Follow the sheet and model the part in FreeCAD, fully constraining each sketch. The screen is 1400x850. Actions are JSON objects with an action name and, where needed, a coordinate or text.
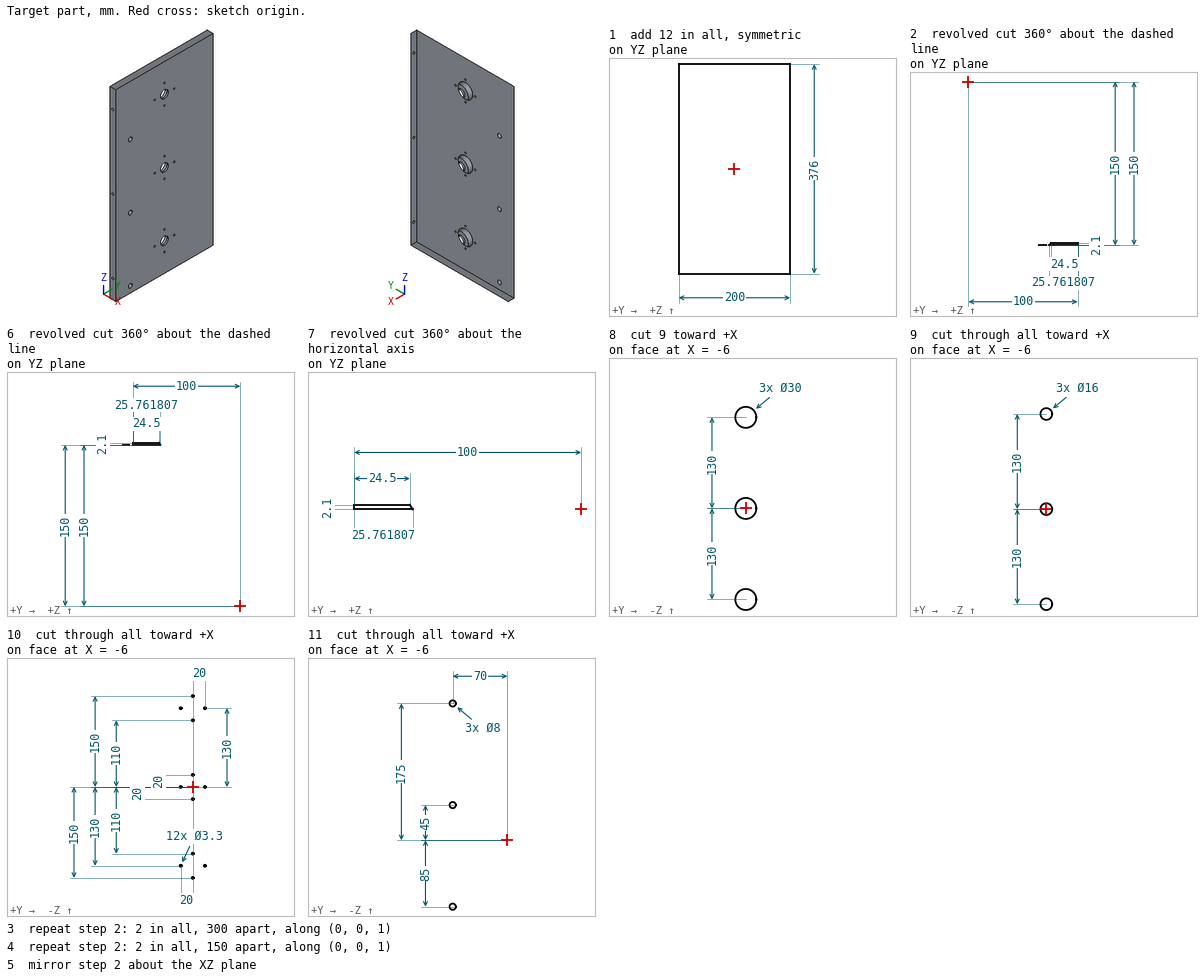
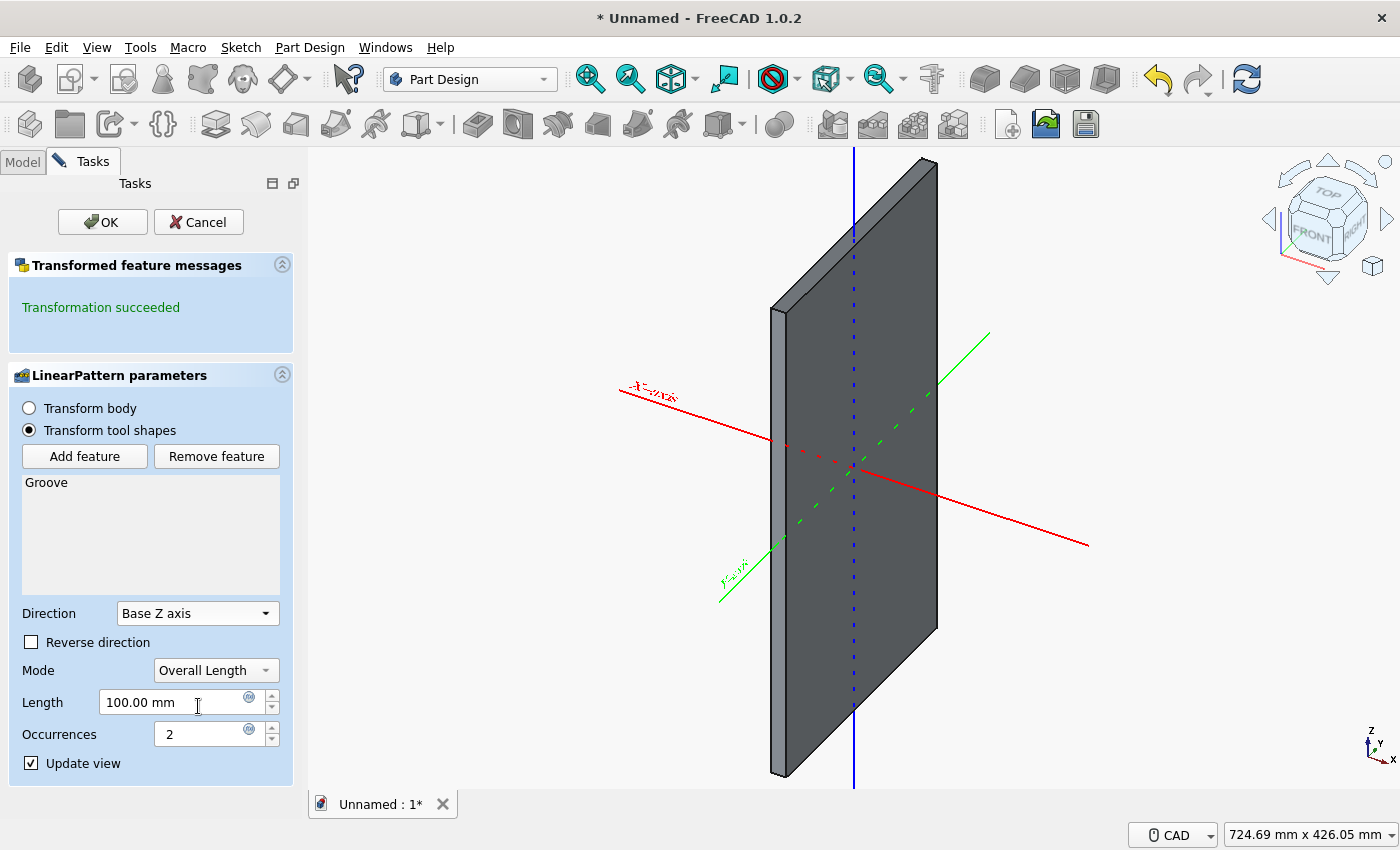
{"action": "left_click", "coordinate": [217, 670]}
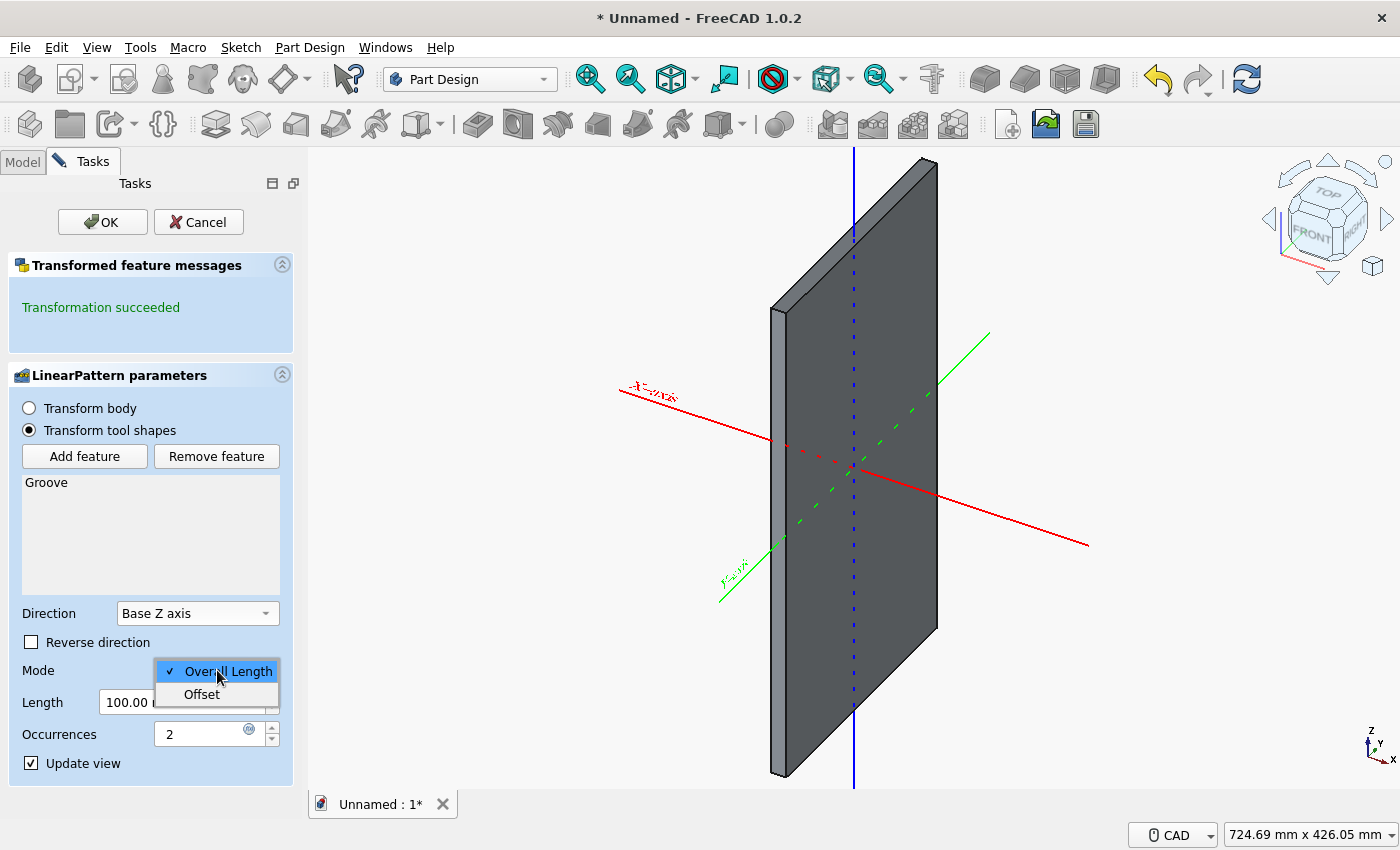
{"action": "left_click", "coordinate": [216, 694]}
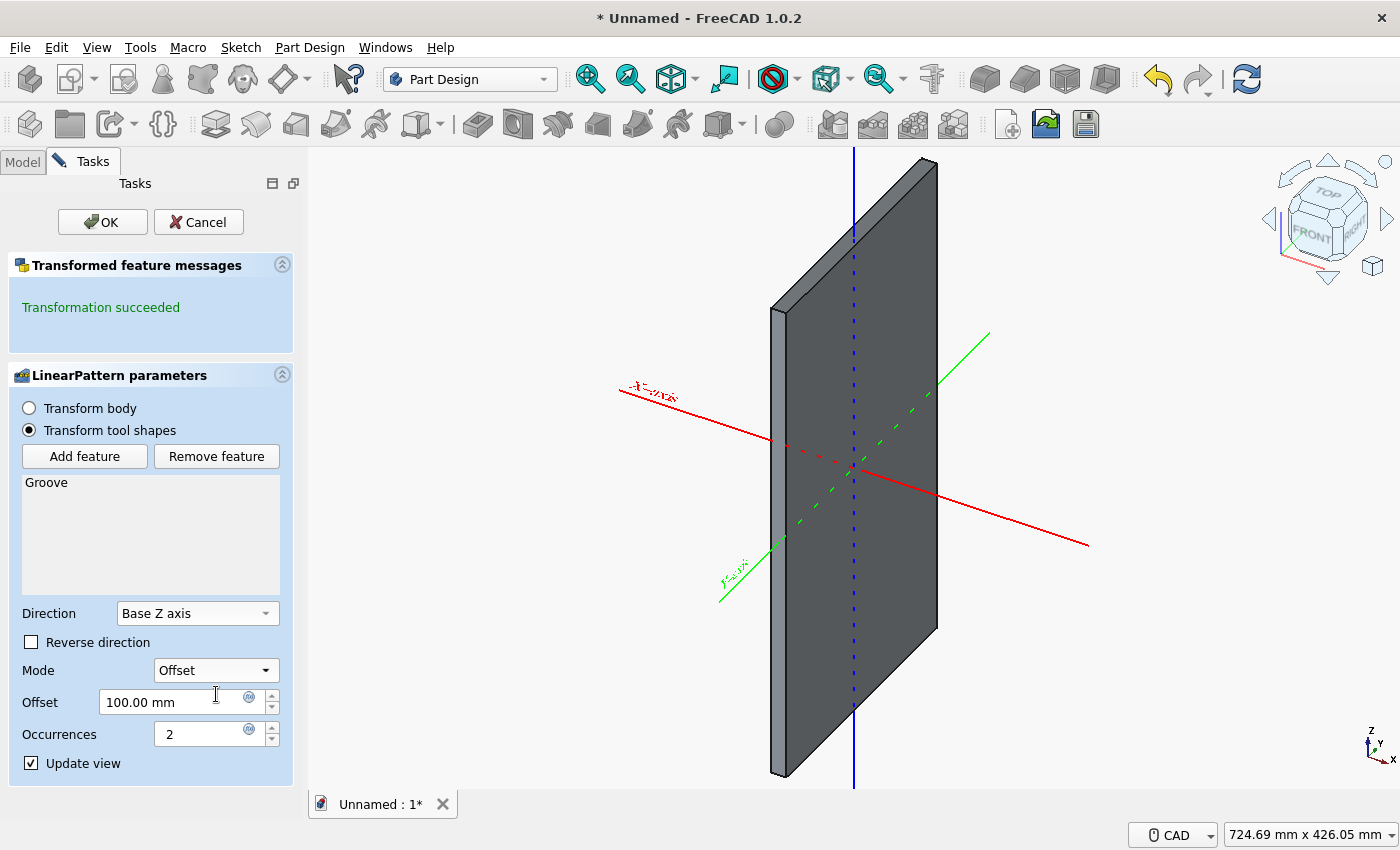
{"action": "triple_click", "coordinate": [182, 702]}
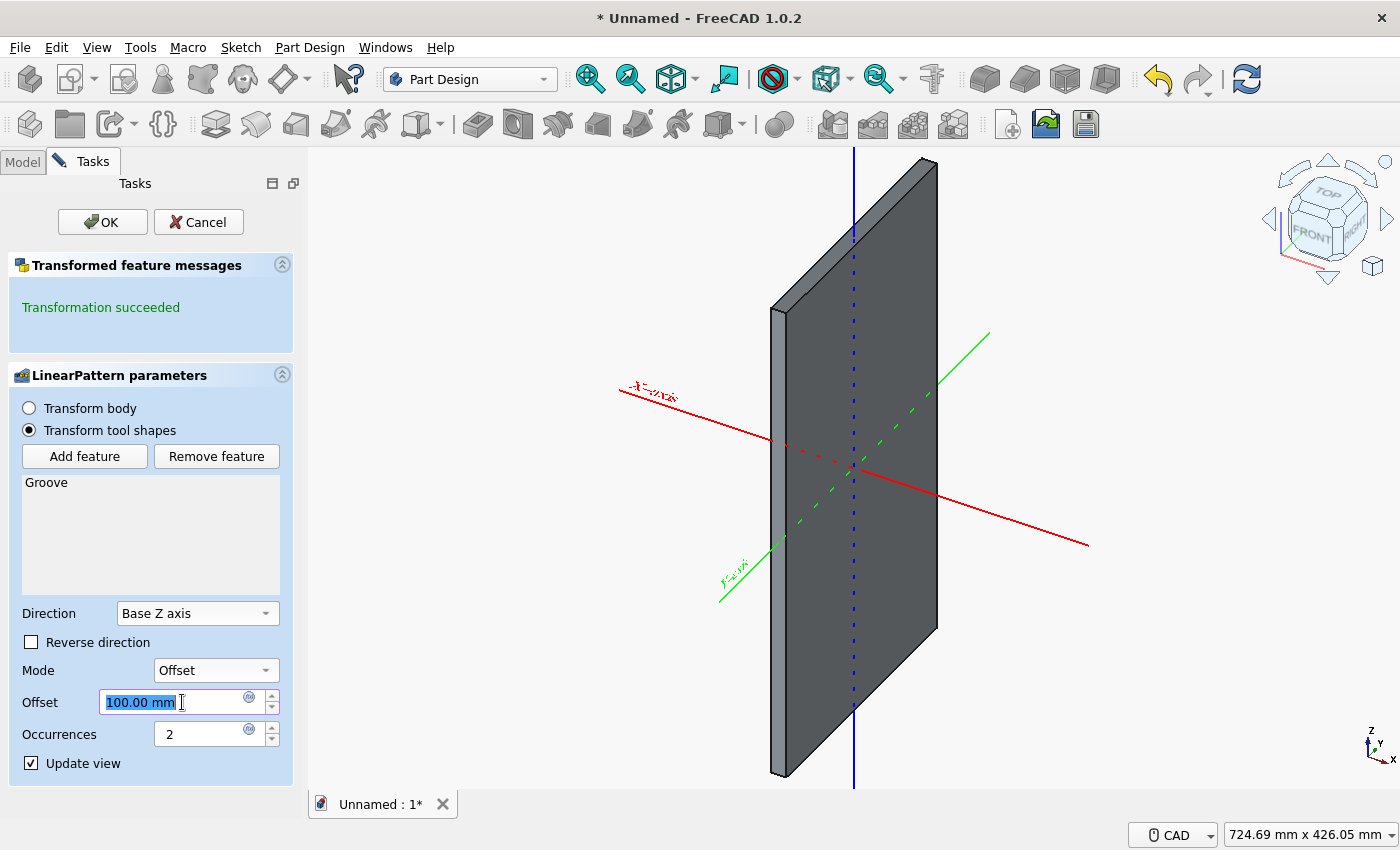
{"action": "type", "text": "300"}
{"action": "key", "text": "Tab"}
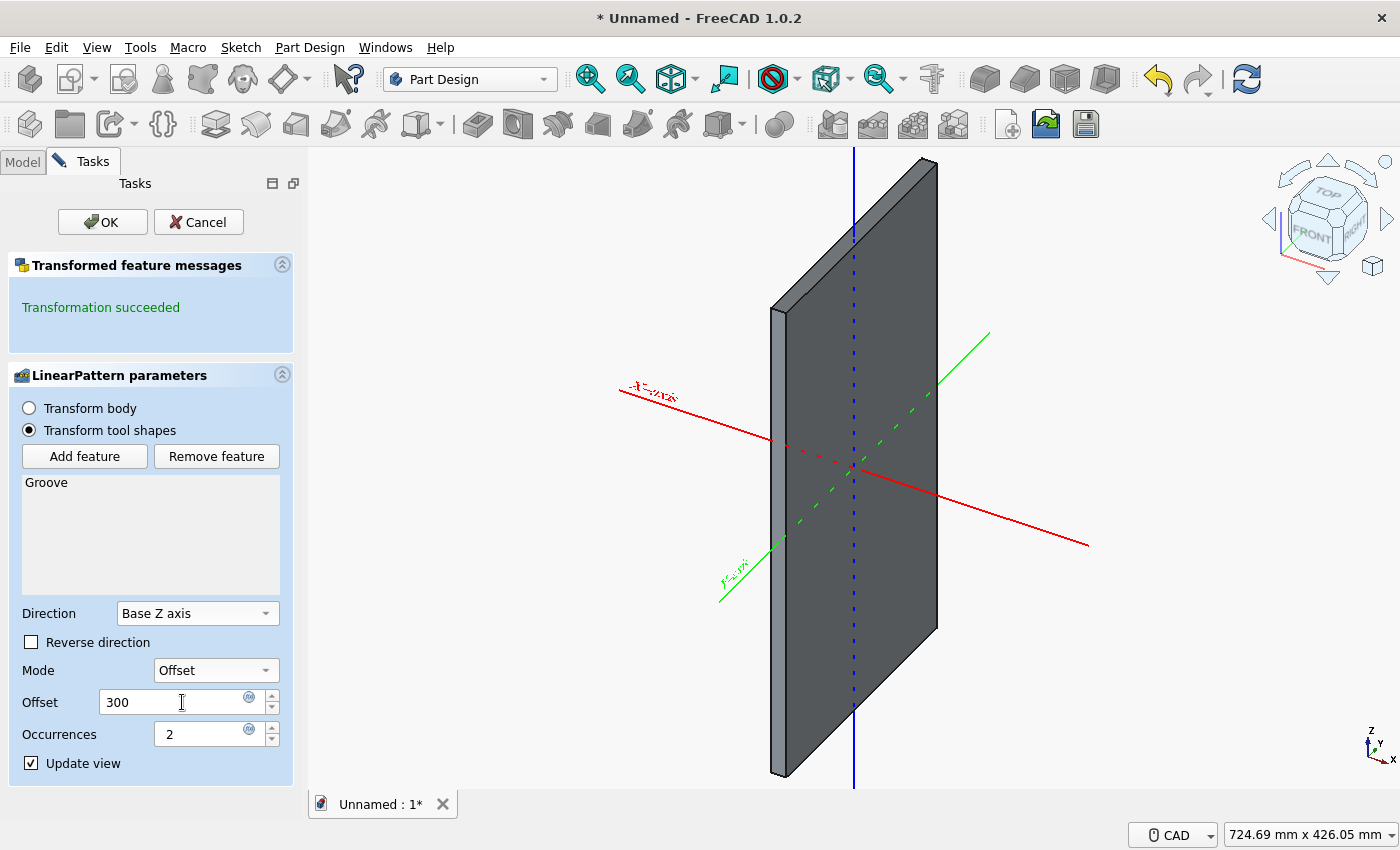
{"action": "triple_click", "coordinate": [209, 734]}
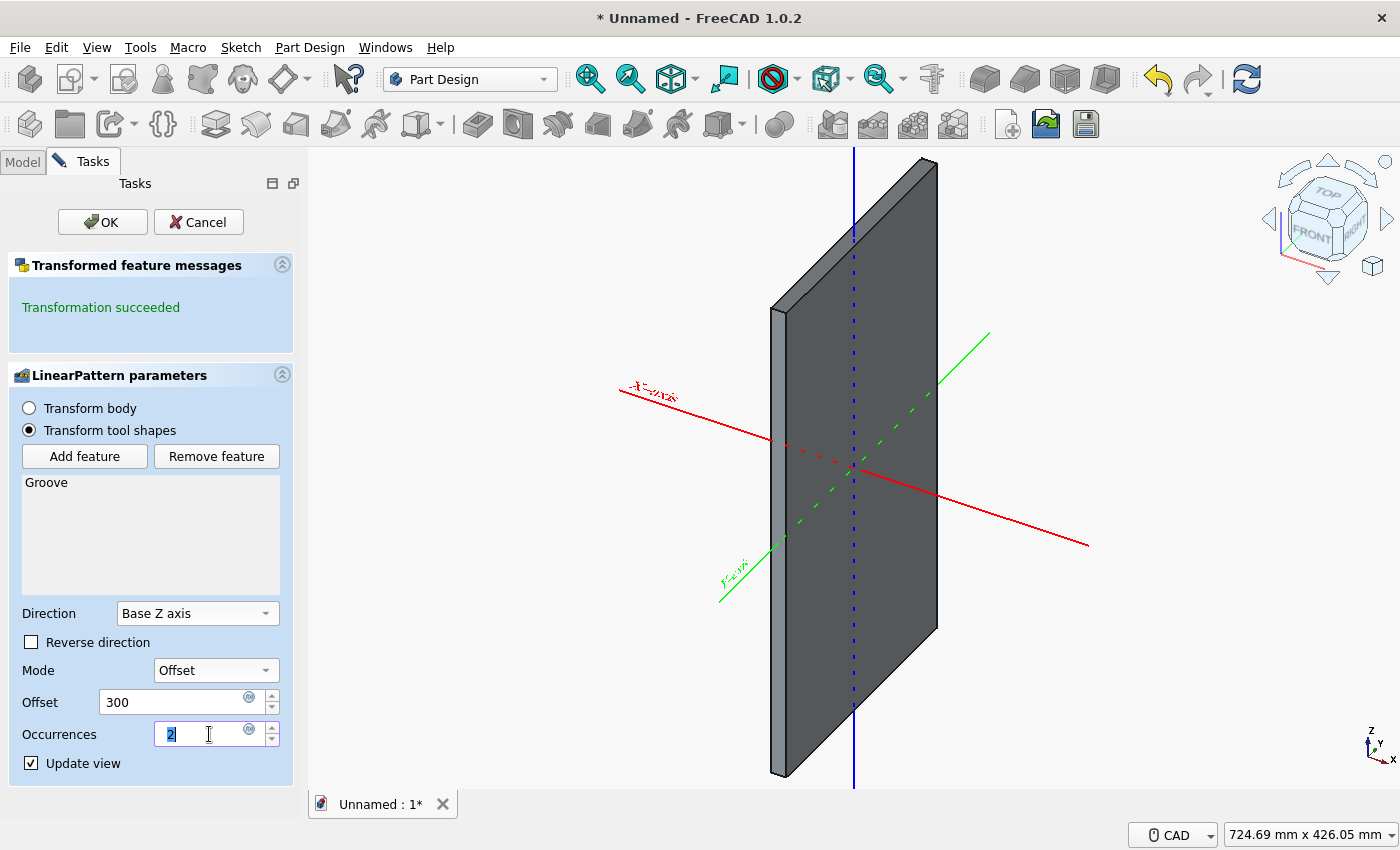
{"action": "type", "text": "2"}
{"action": "key", "text": "Tab"}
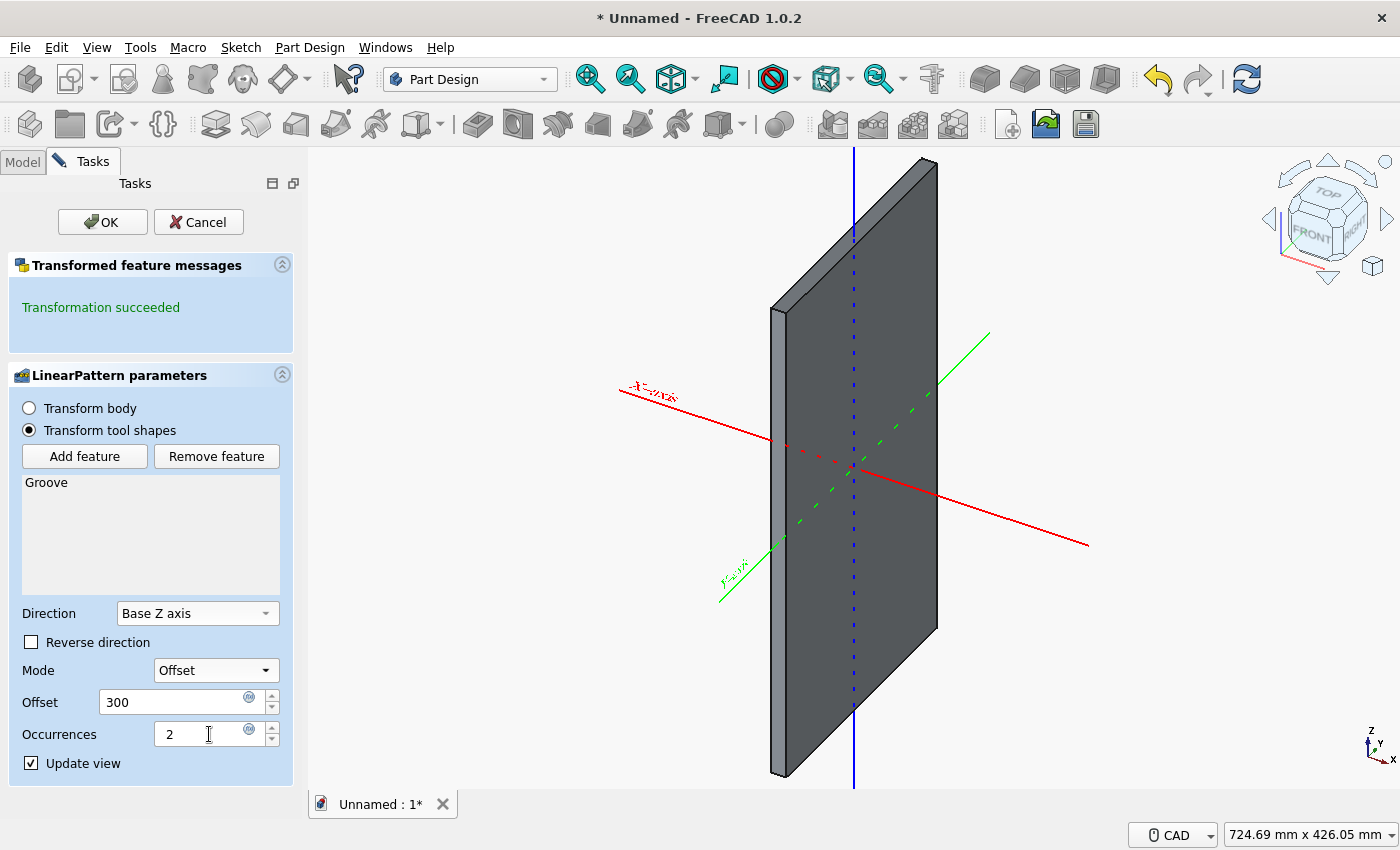
{"action": "left_click", "coordinate": [103, 222]}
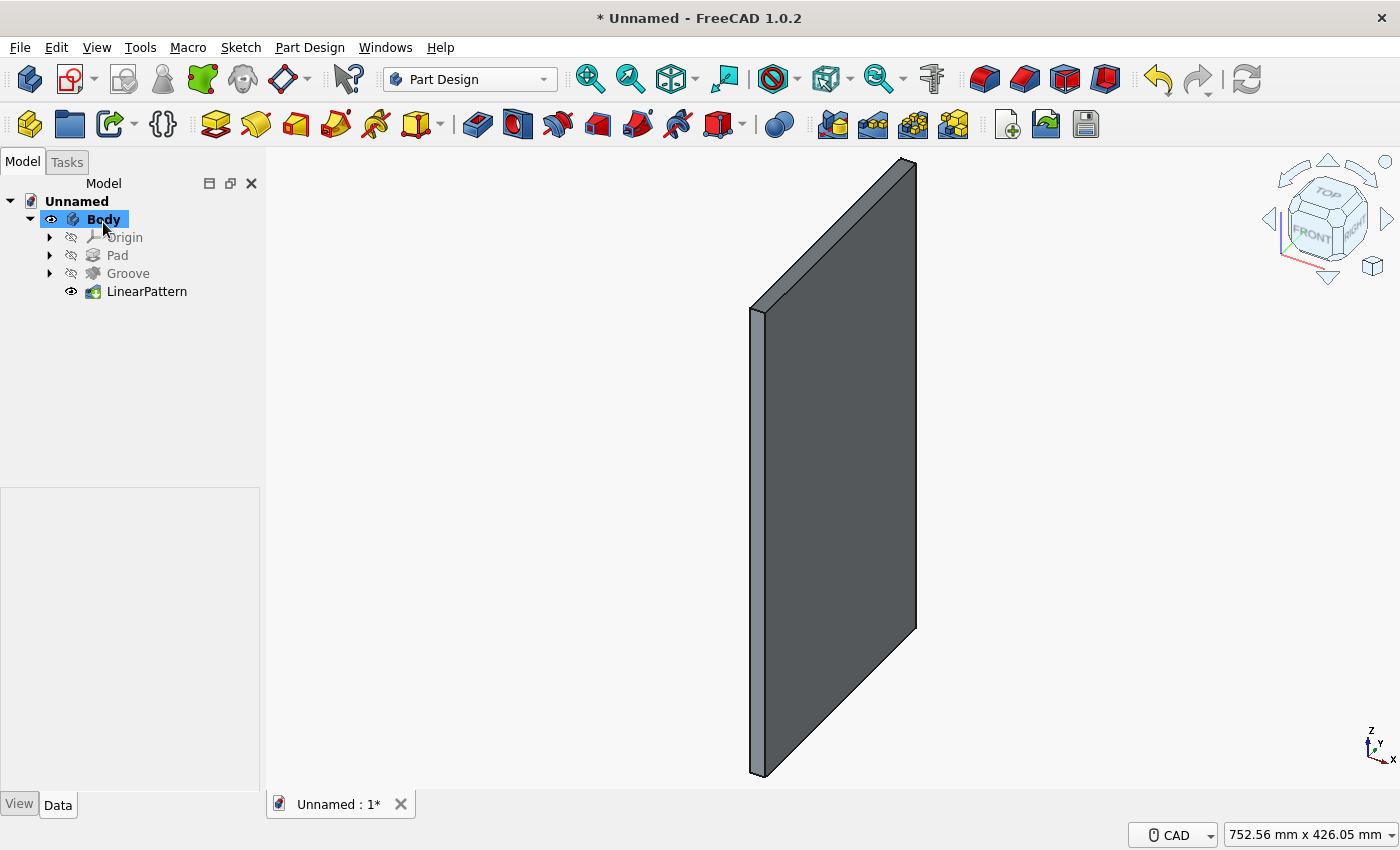
{"action": "left_click", "coordinate": [116, 273]}